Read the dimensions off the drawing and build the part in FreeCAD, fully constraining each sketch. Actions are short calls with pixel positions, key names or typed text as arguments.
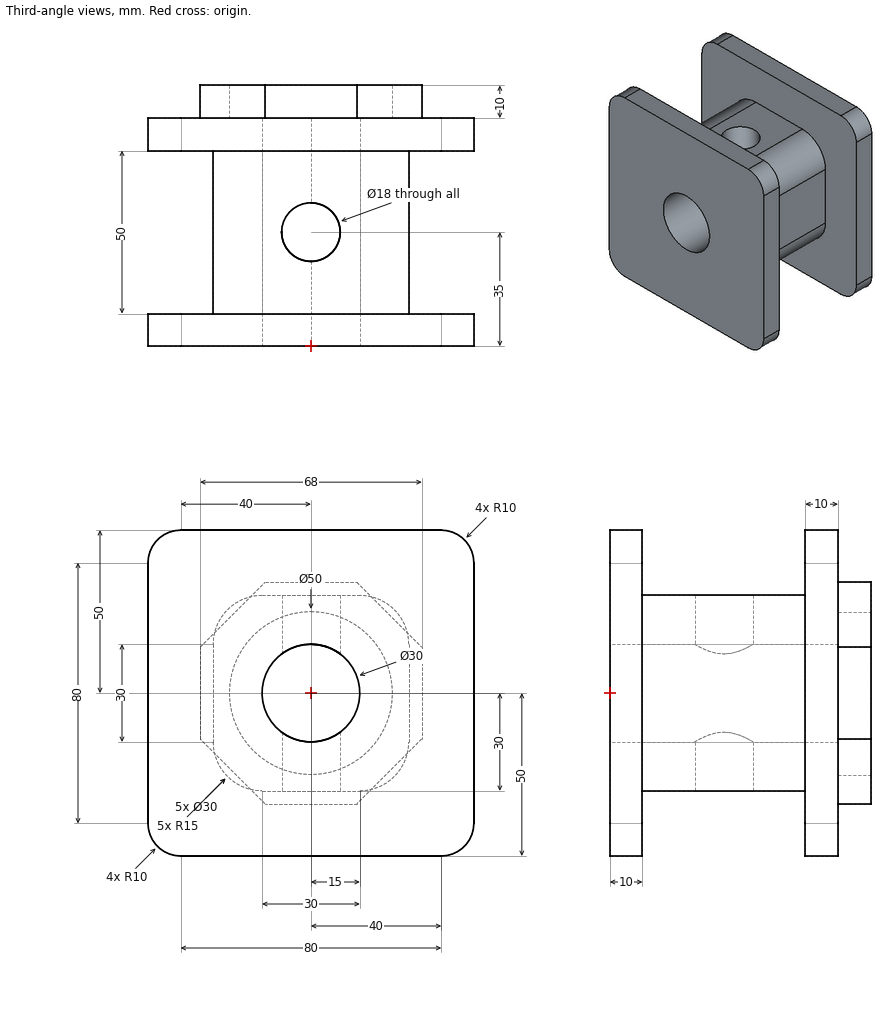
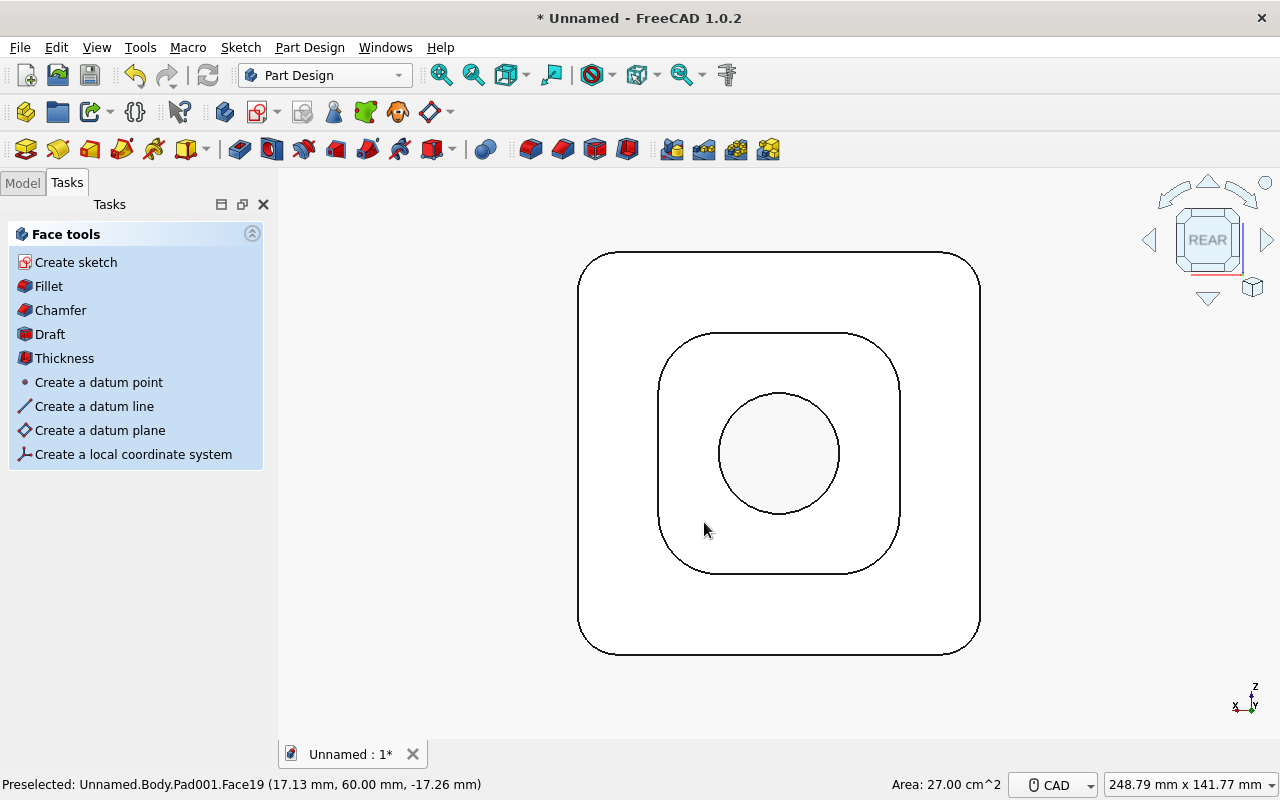
click(258, 112)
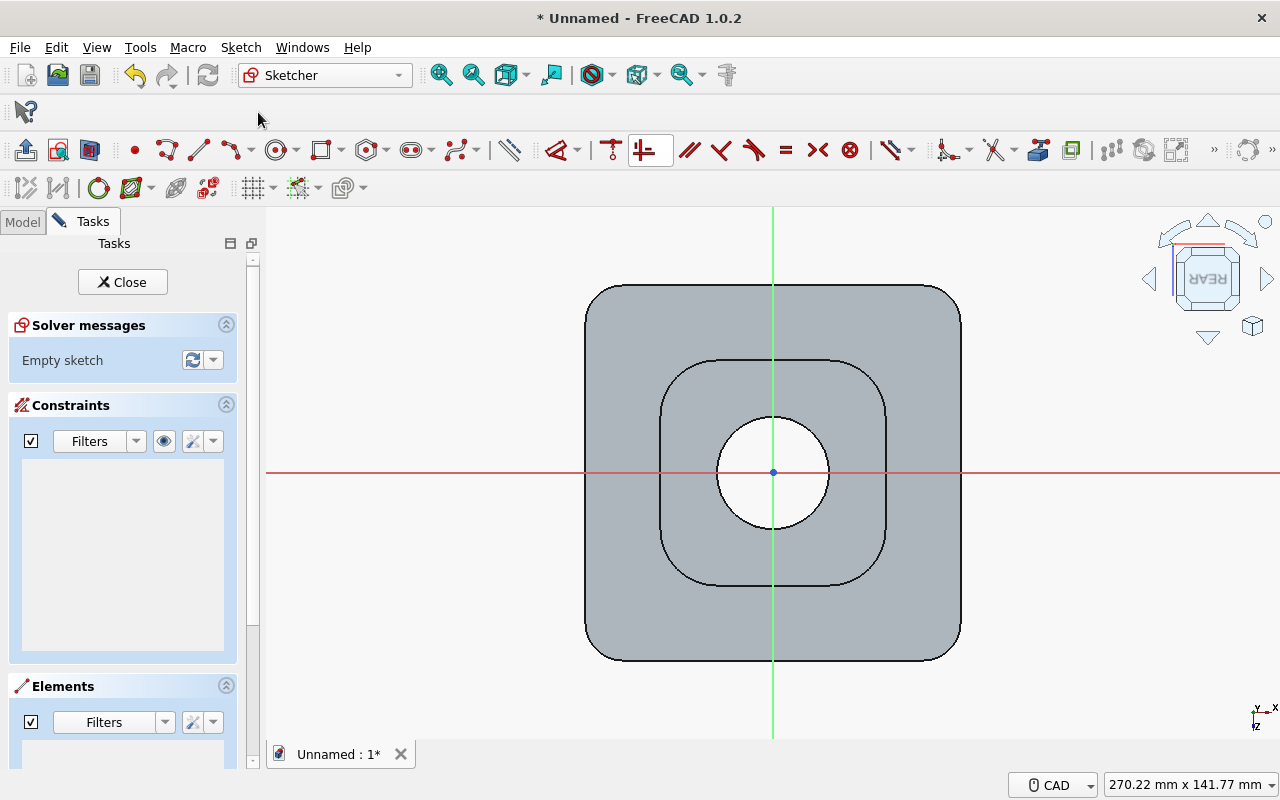
click(200, 150)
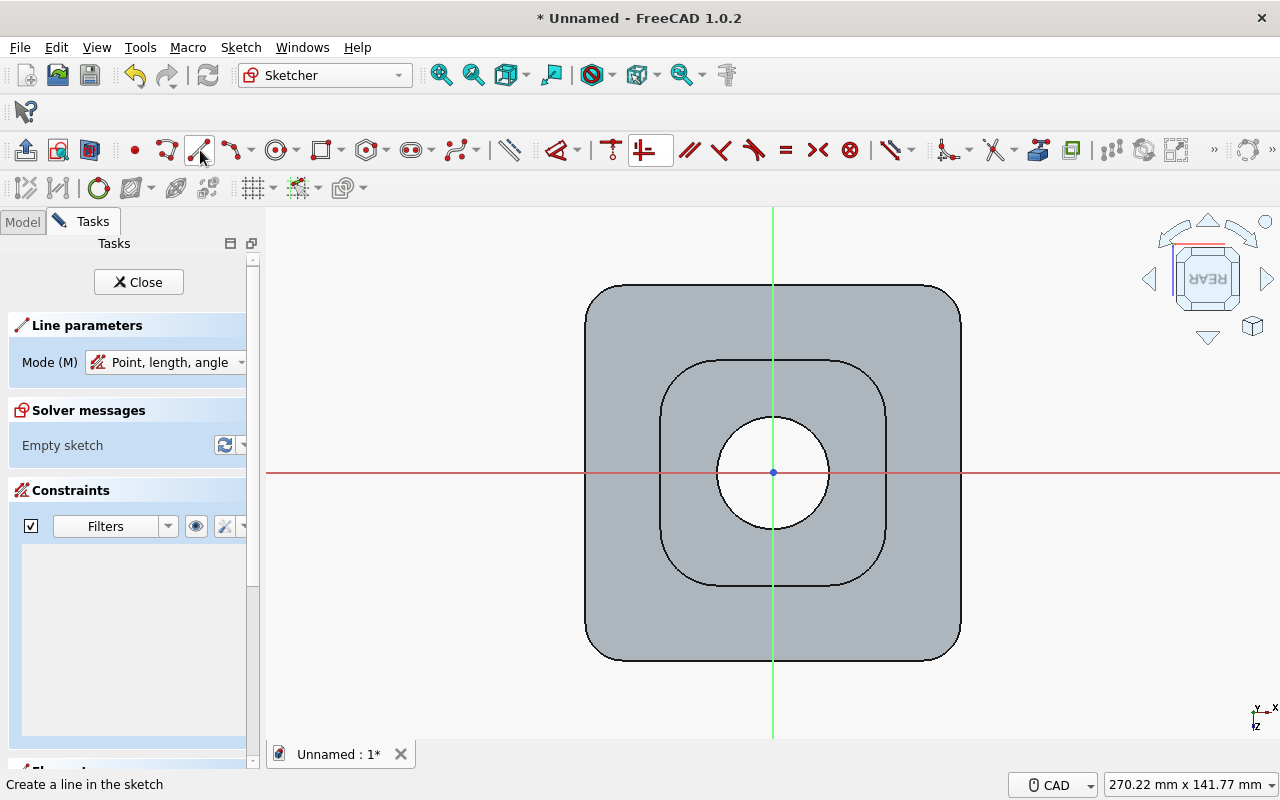
click(623, 661)
click(923, 661)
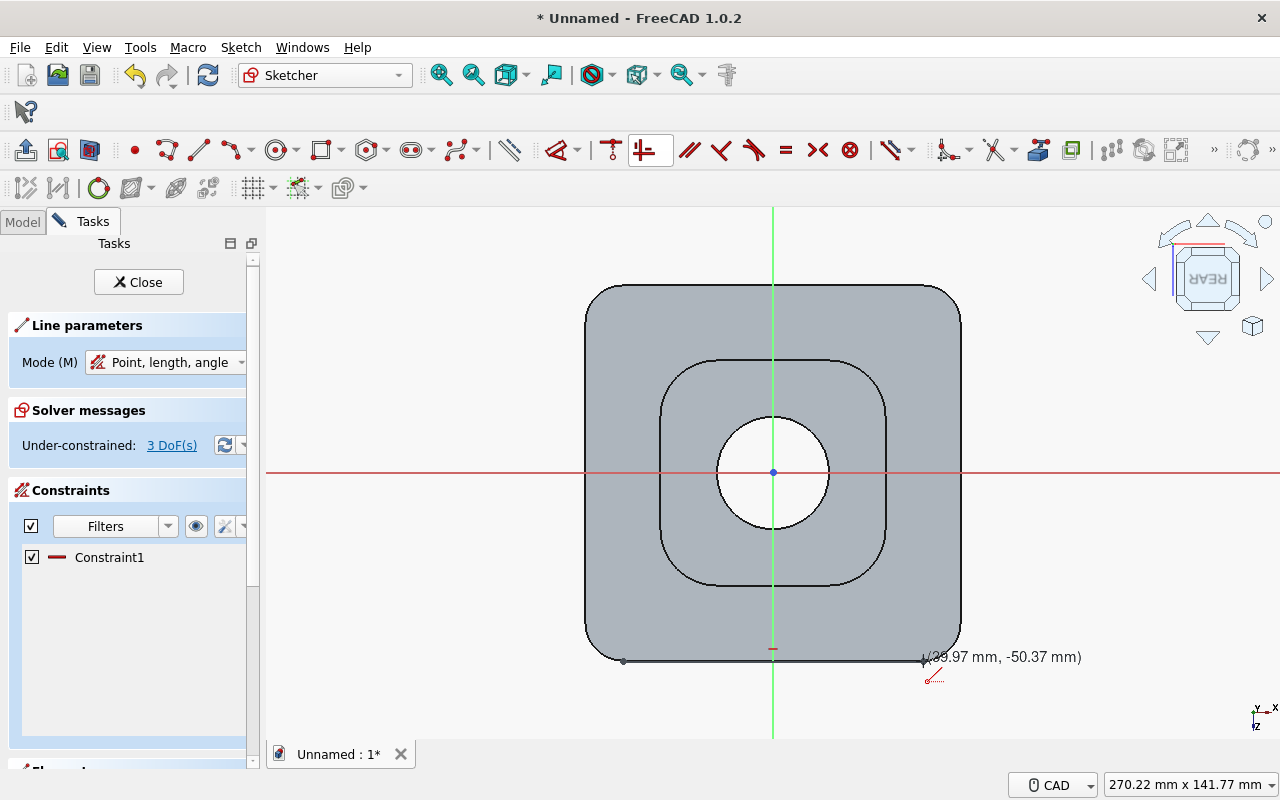
click(961, 623)
click(961, 323)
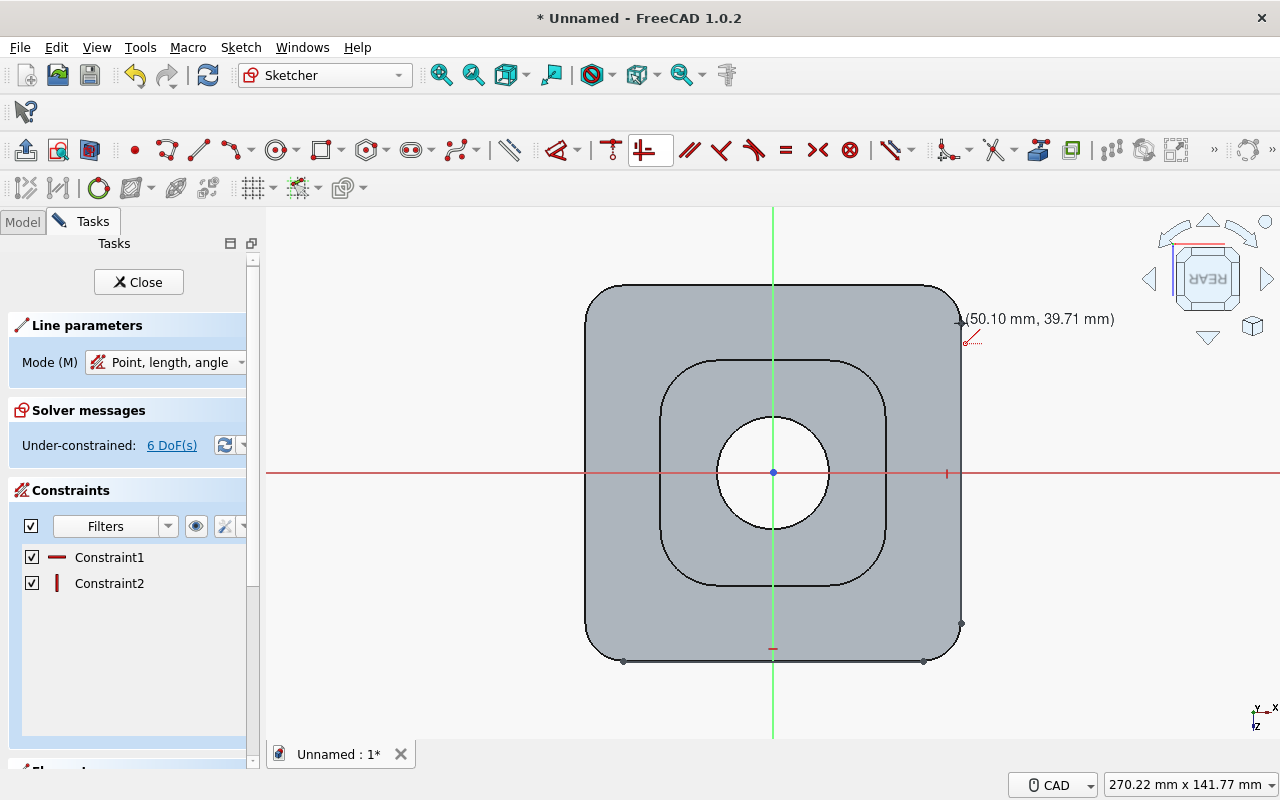
click(923, 285)
click(623, 285)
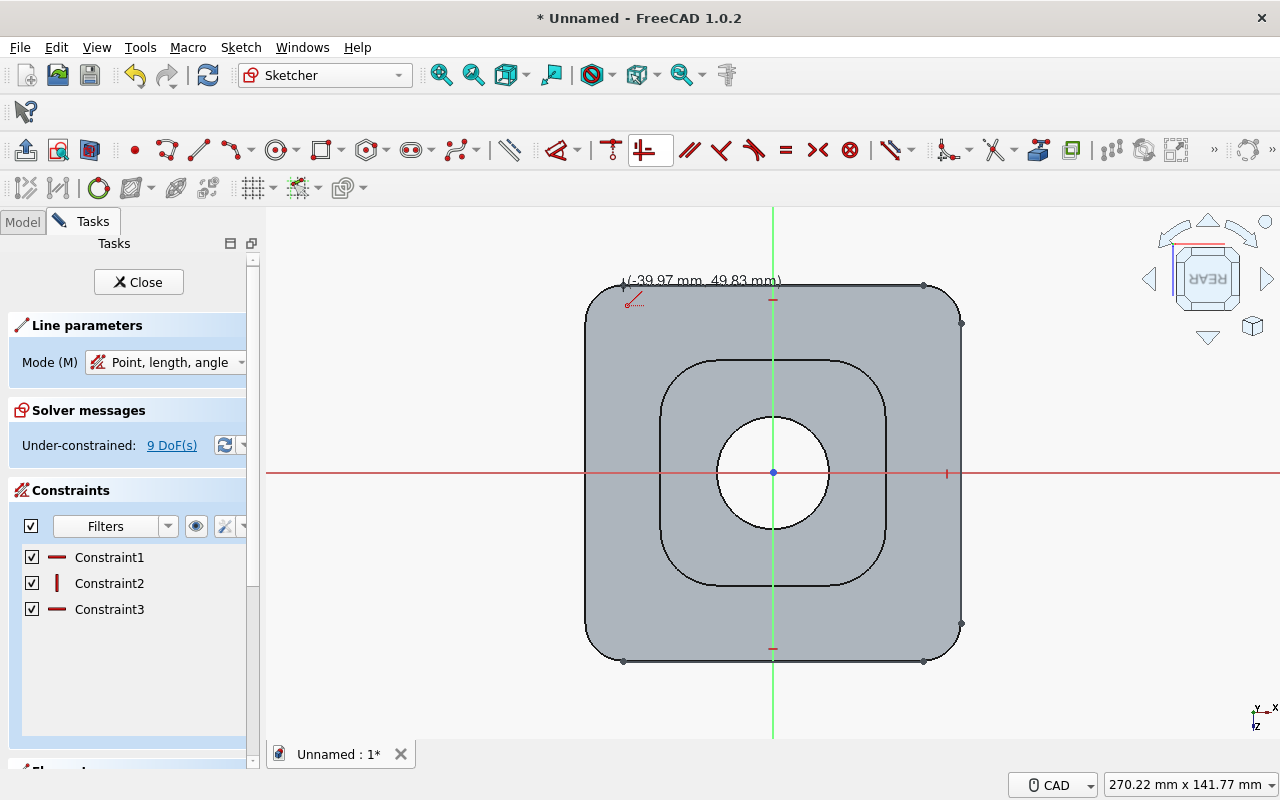
click(585, 323)
click(585, 623)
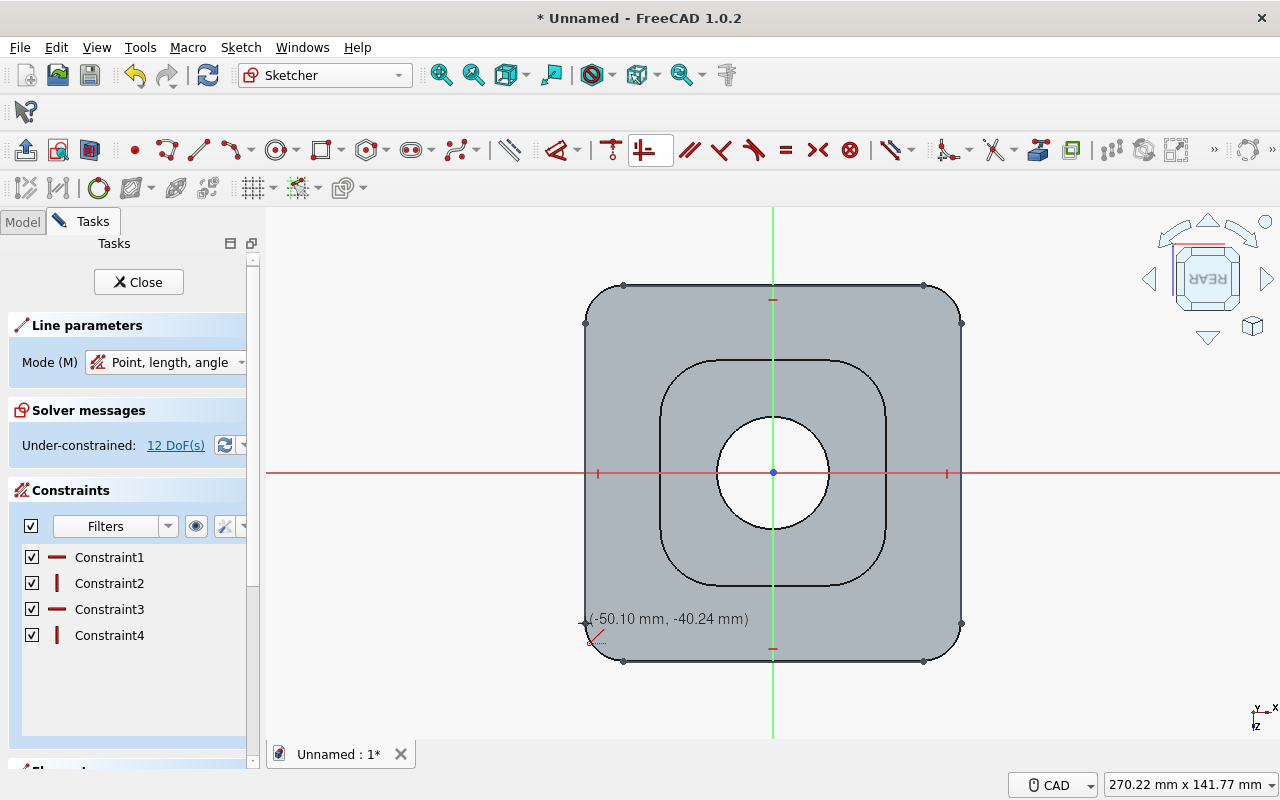
click(232, 150)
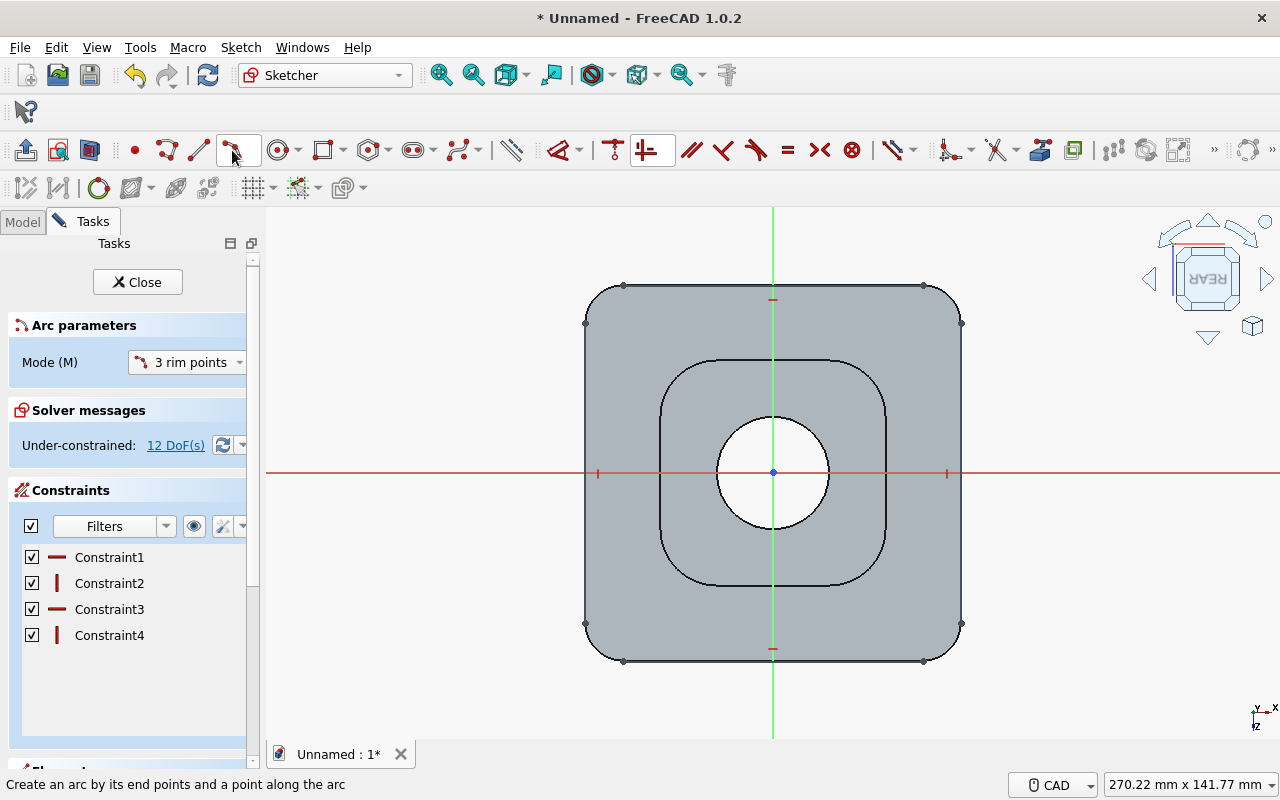
click(923, 662)
click(961, 624)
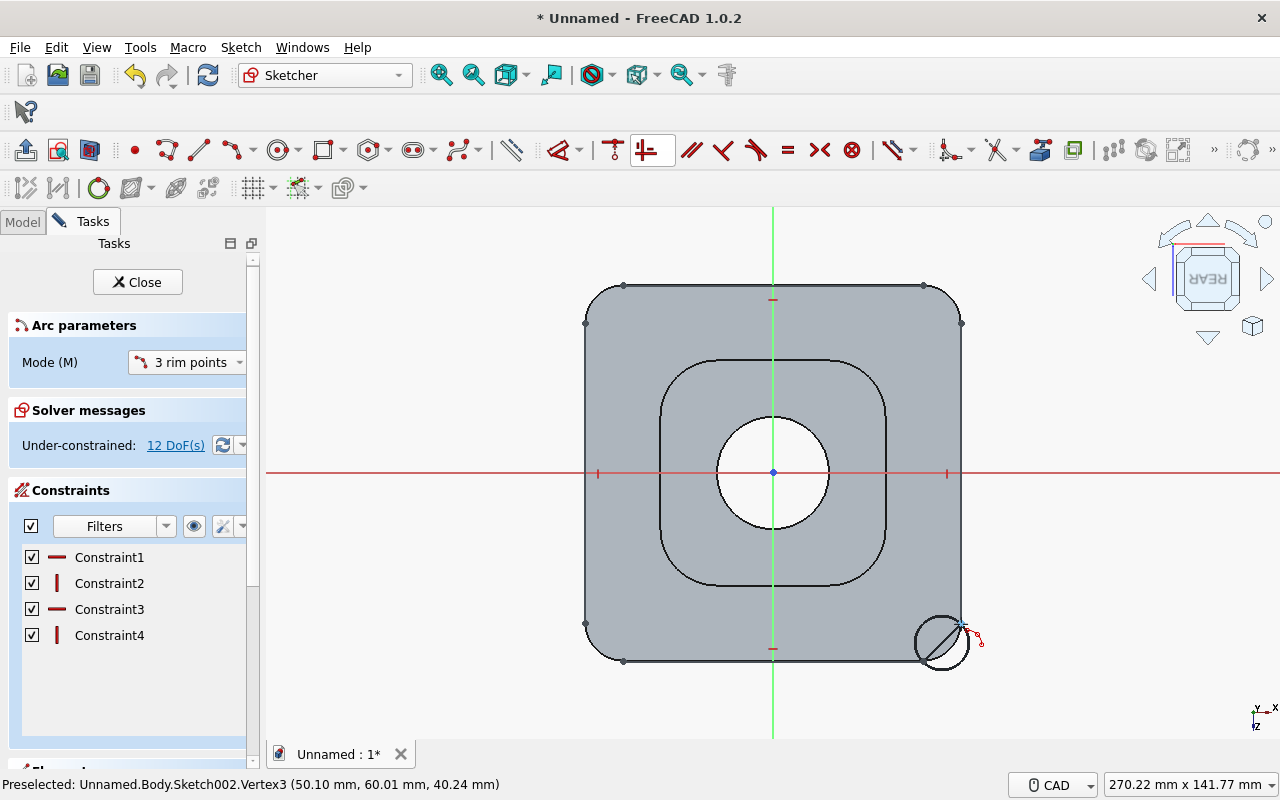
scroll(950, 650, up, 2)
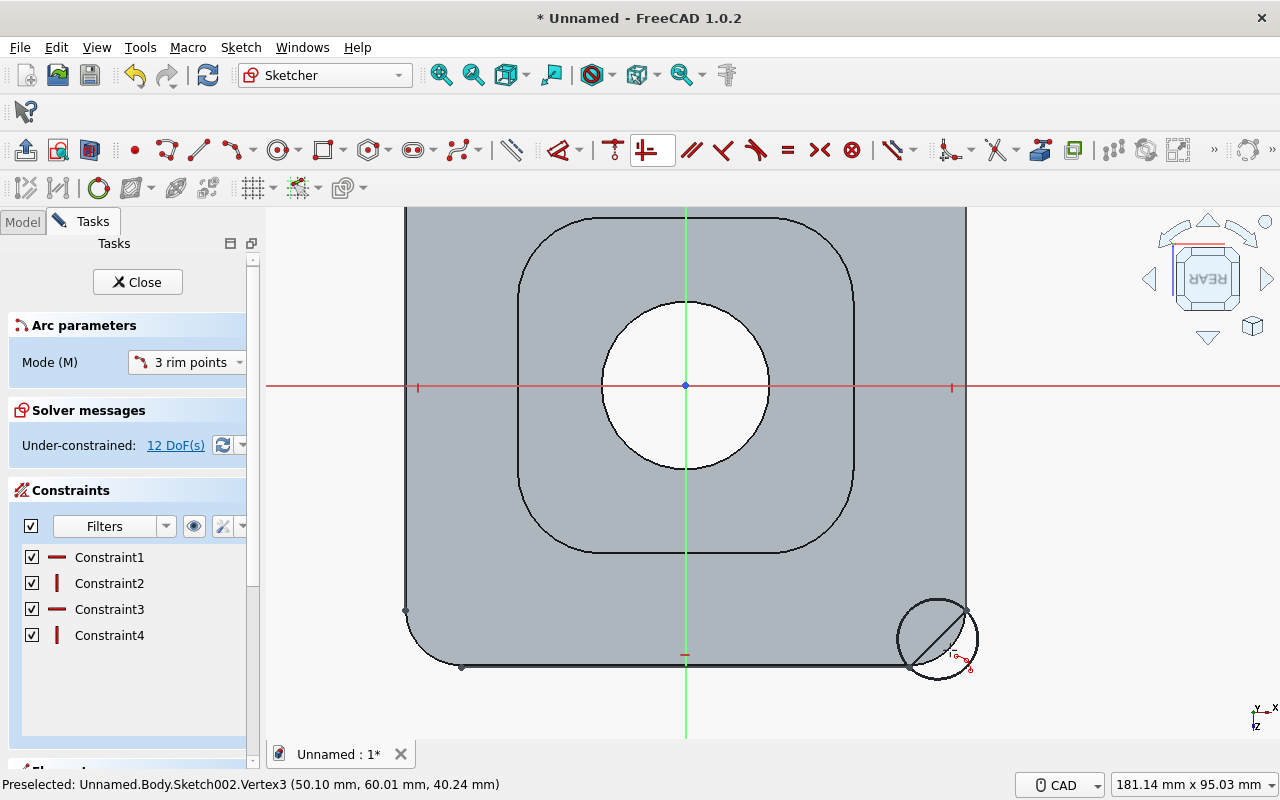
click(949, 649)